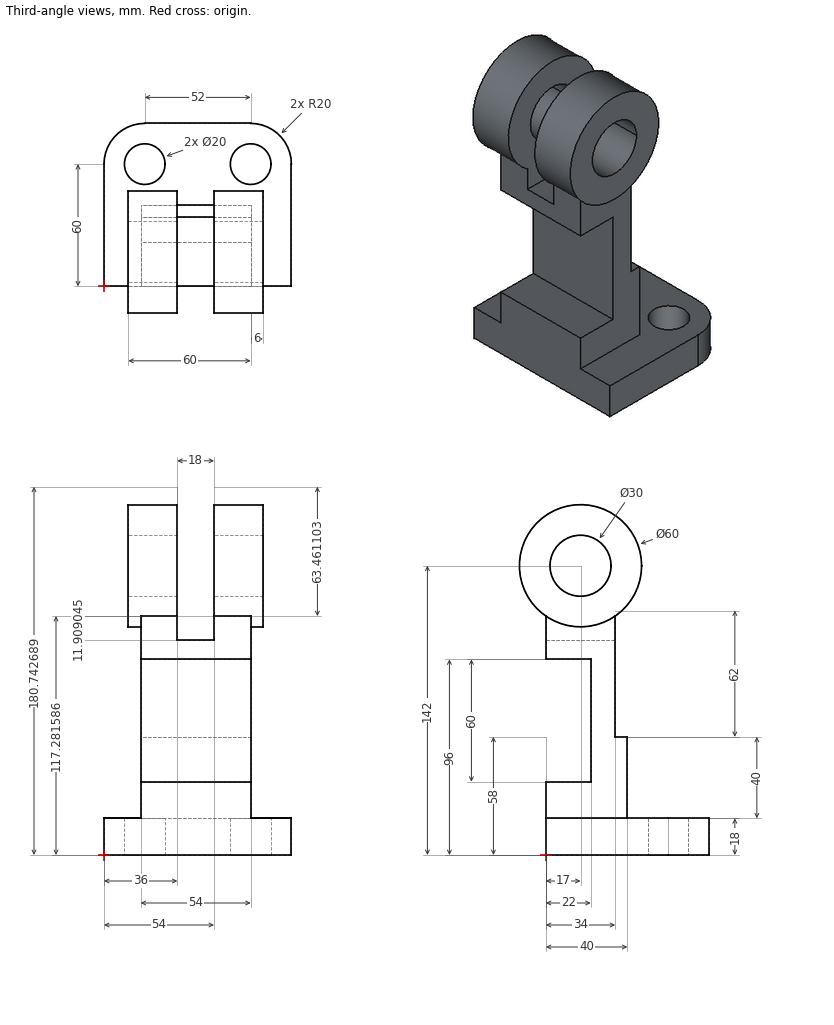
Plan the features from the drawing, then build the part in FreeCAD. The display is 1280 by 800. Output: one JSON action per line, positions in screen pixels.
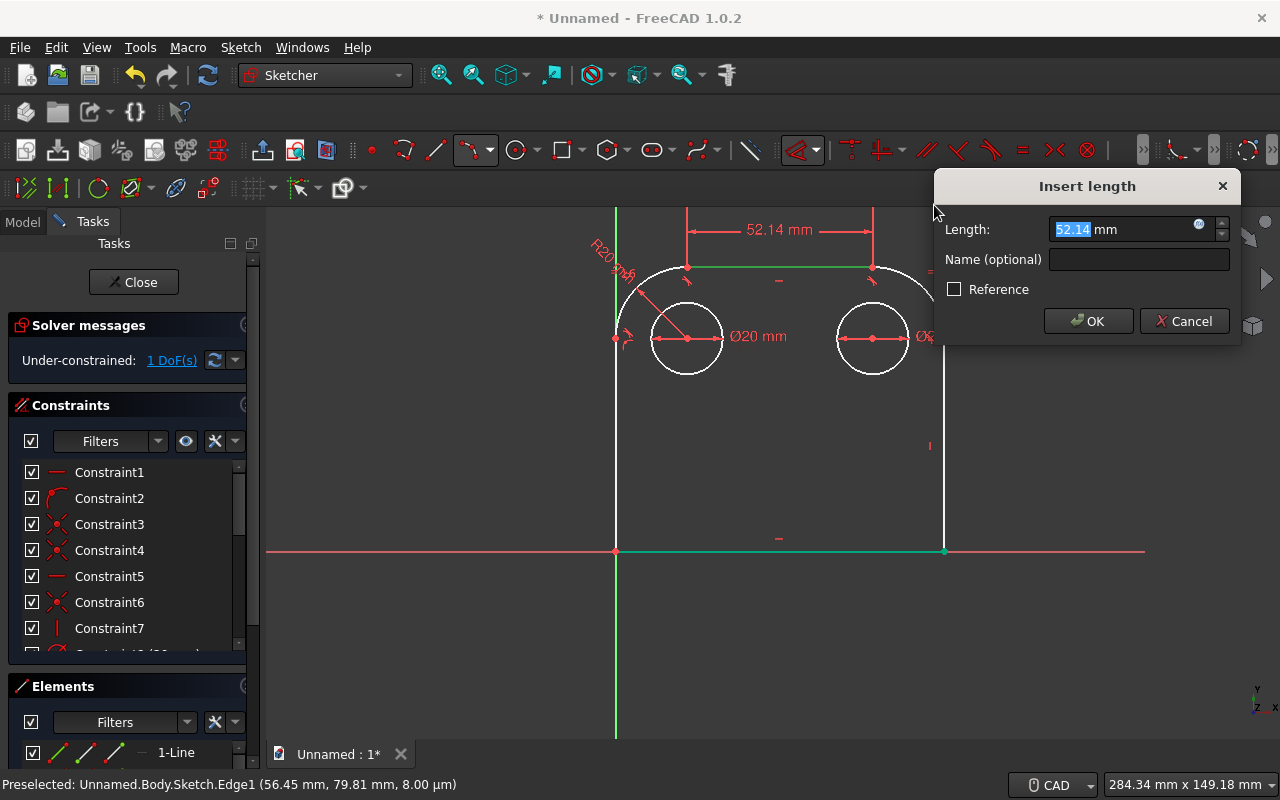
{"action": "type", "text": "52"}
{"action": "key", "text": "Return"}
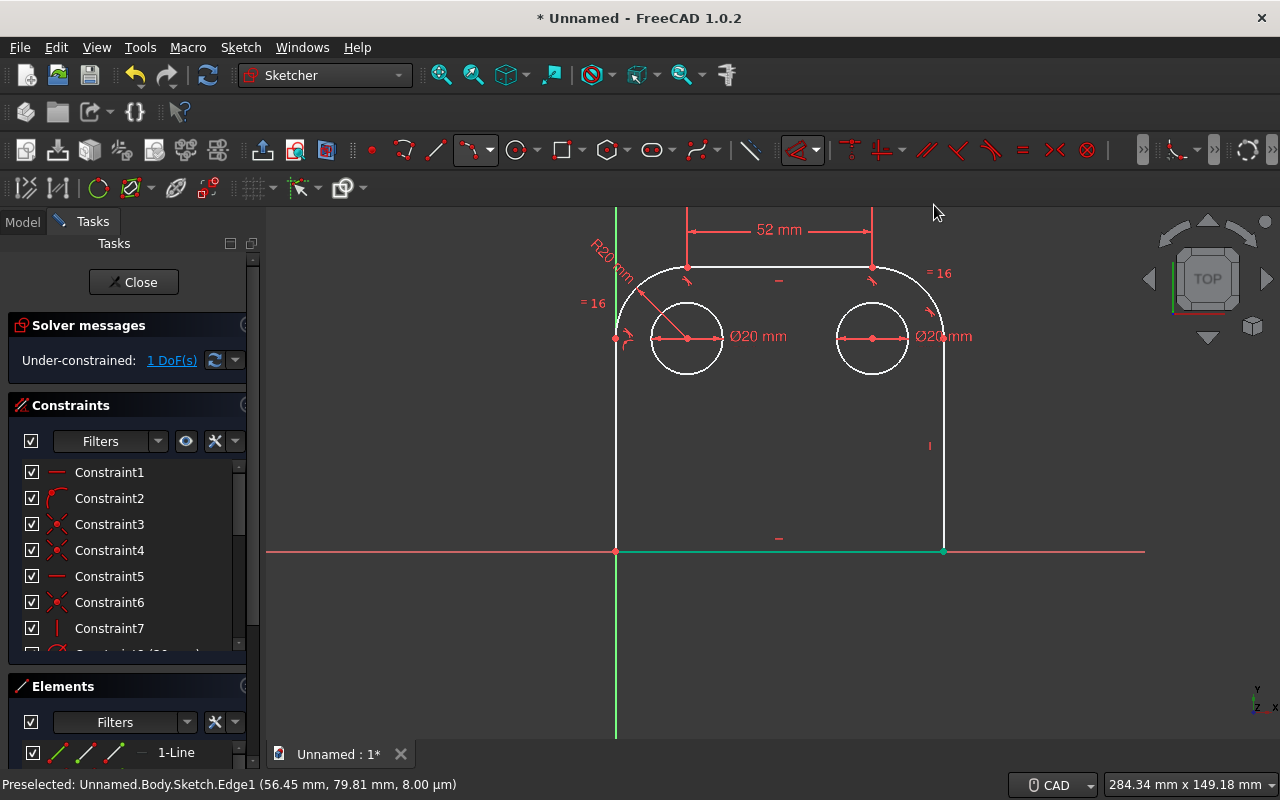
{"action": "left_click", "coordinate": [616, 402]}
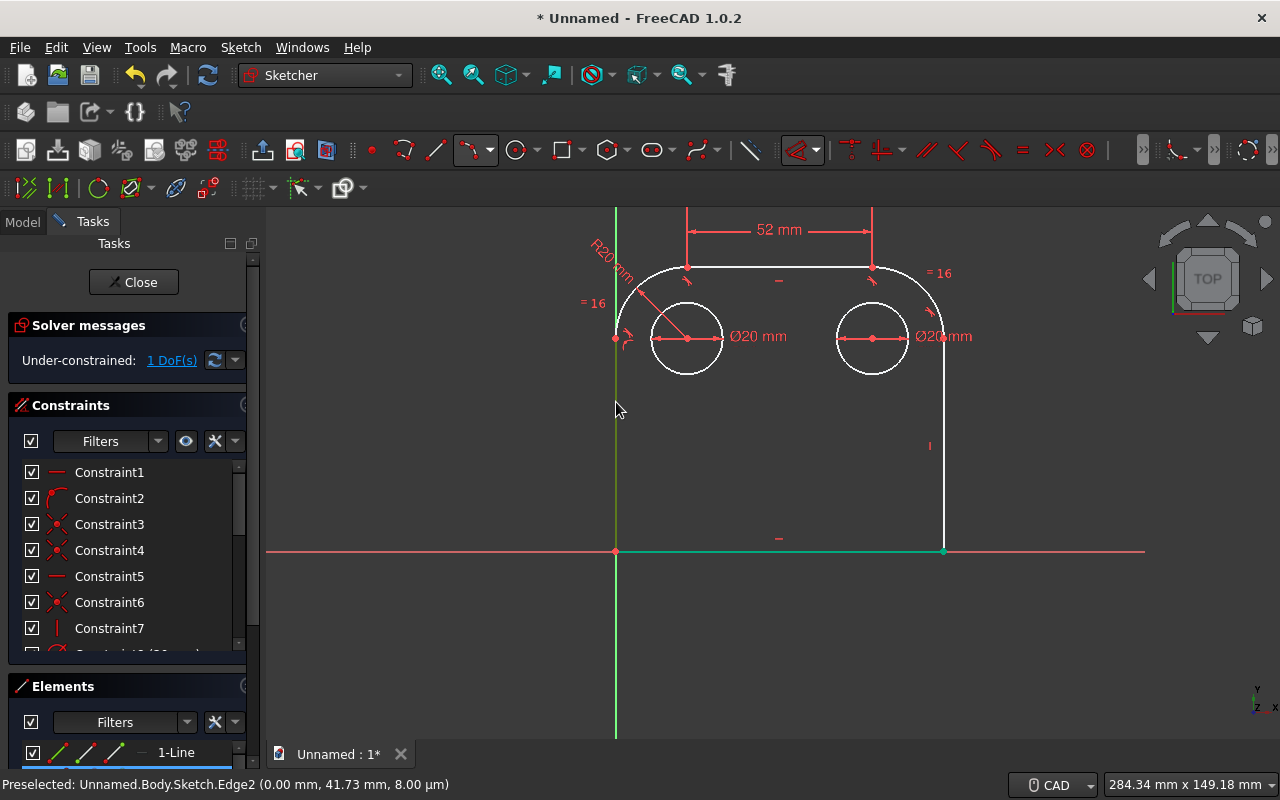
{"action": "key", "text": "i"}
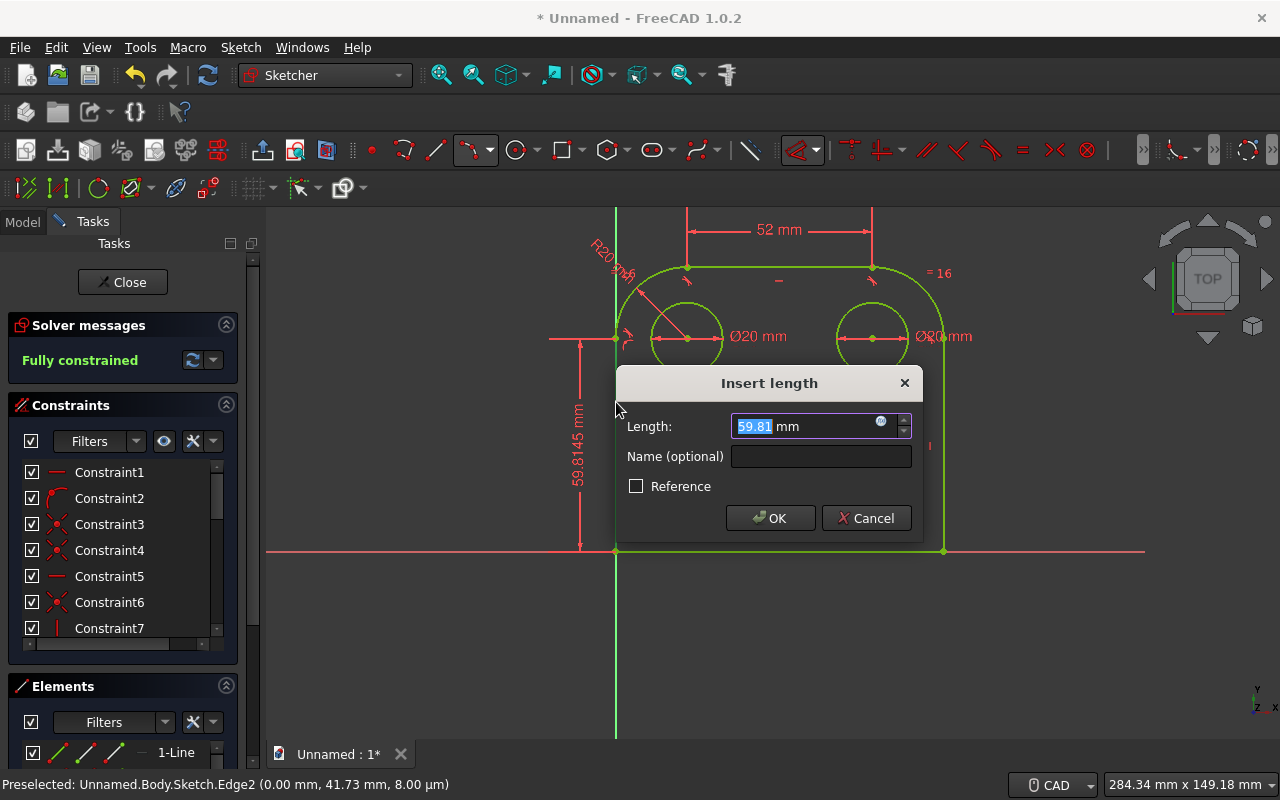
{"action": "type", "text": "60"}
{"action": "key", "text": "Return"}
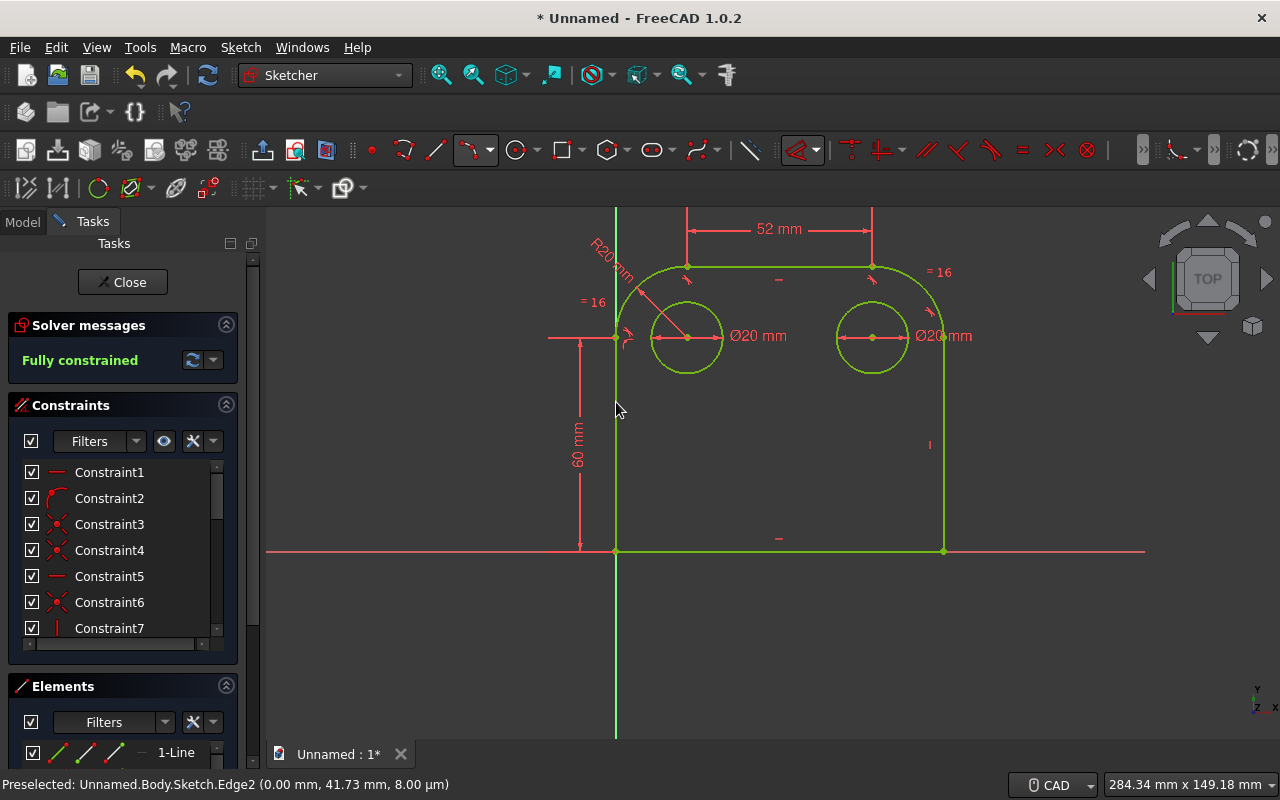
{"action": "left_click", "coordinate": [123, 282]}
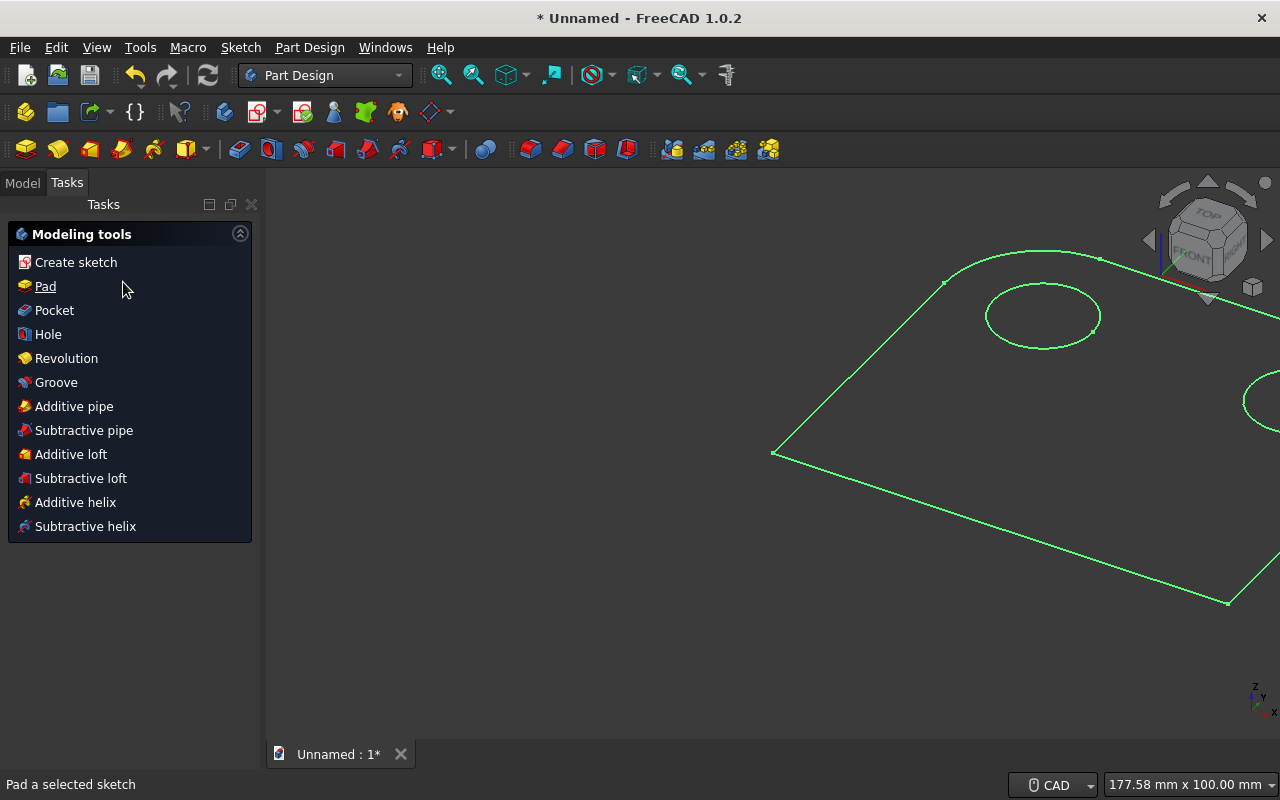
{"action": "left_click", "coordinate": [26, 150]}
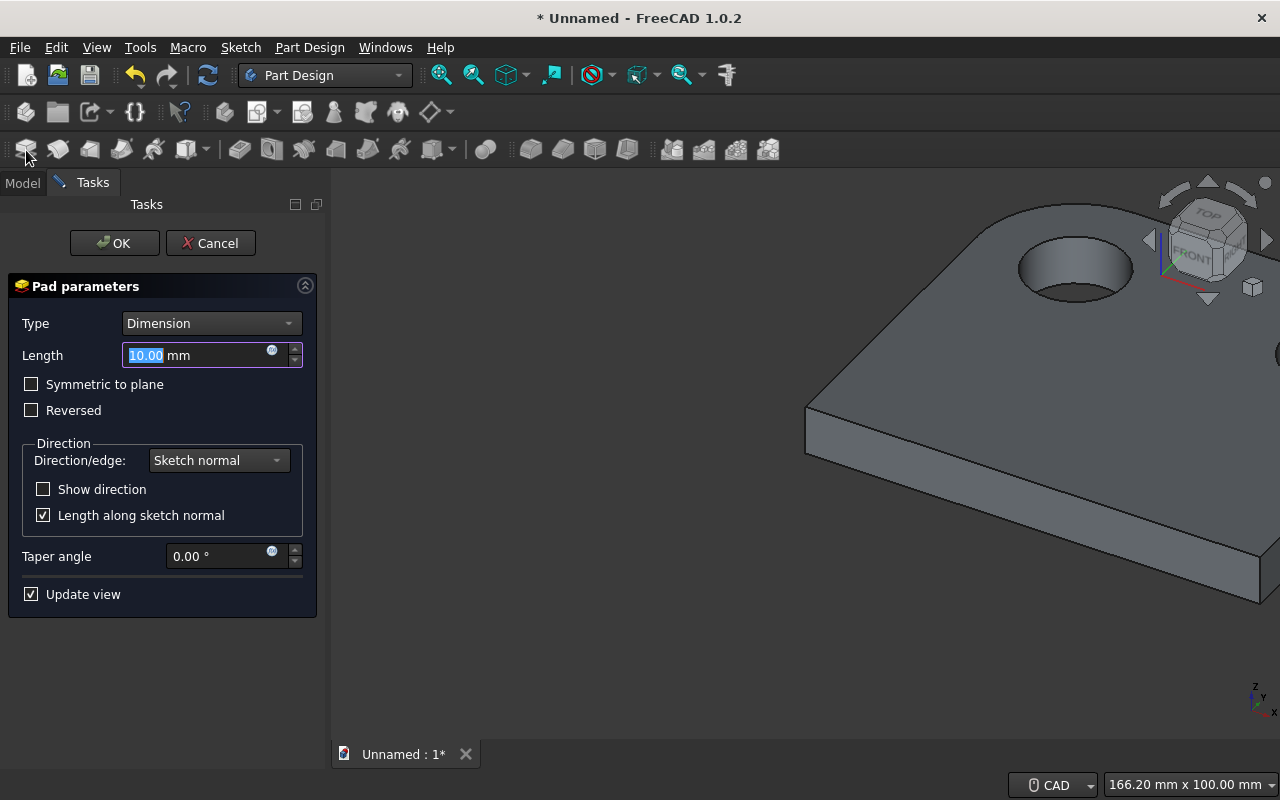
{"action": "type", "text": "18"}
{"action": "key", "text": "Tab"}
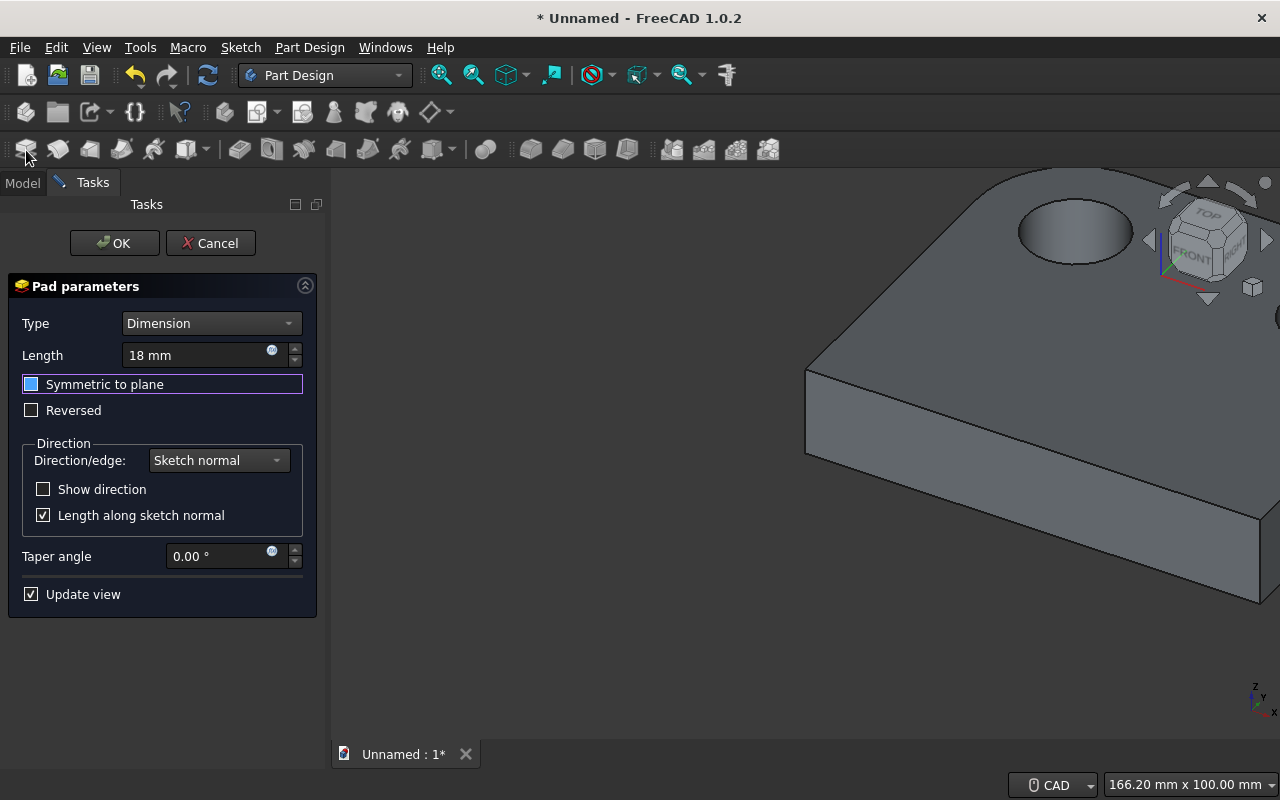
{"action": "left_click", "coordinate": [115, 243]}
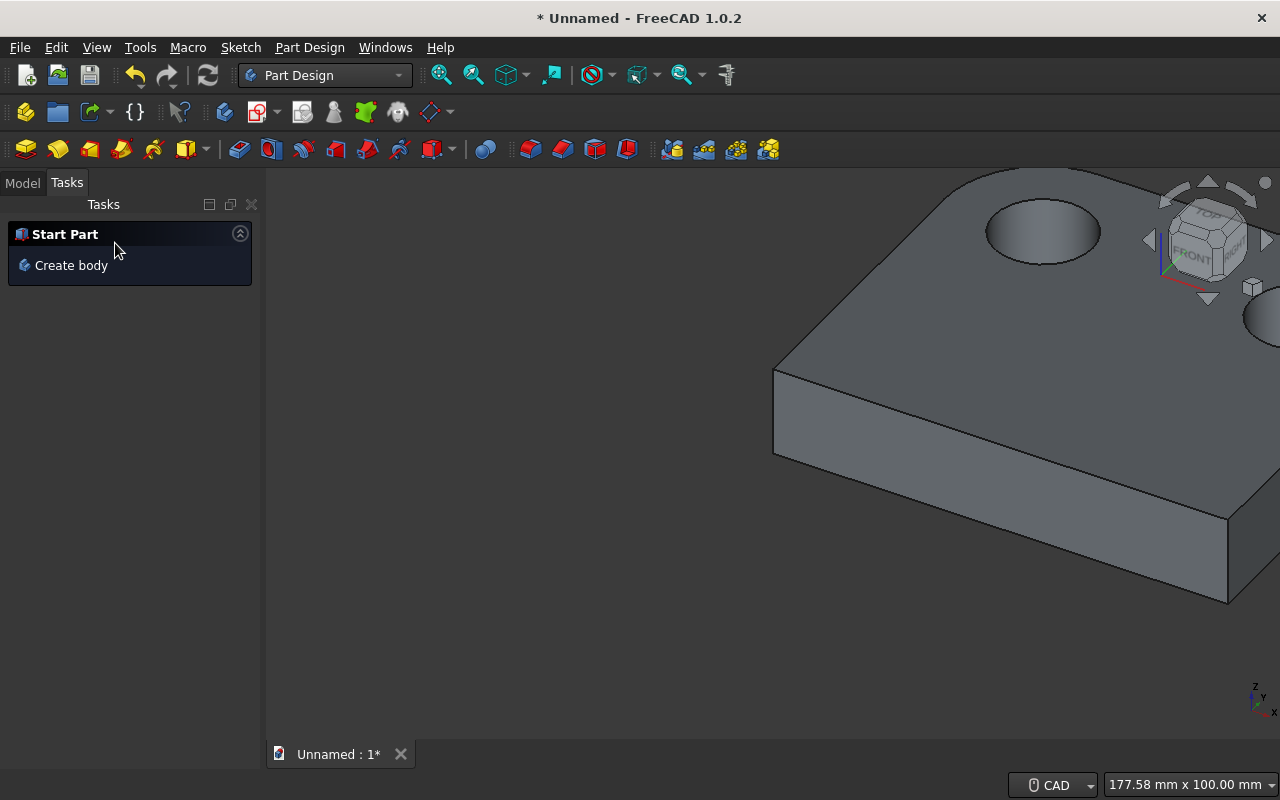
{"action": "left_click", "coordinate": [442, 76]}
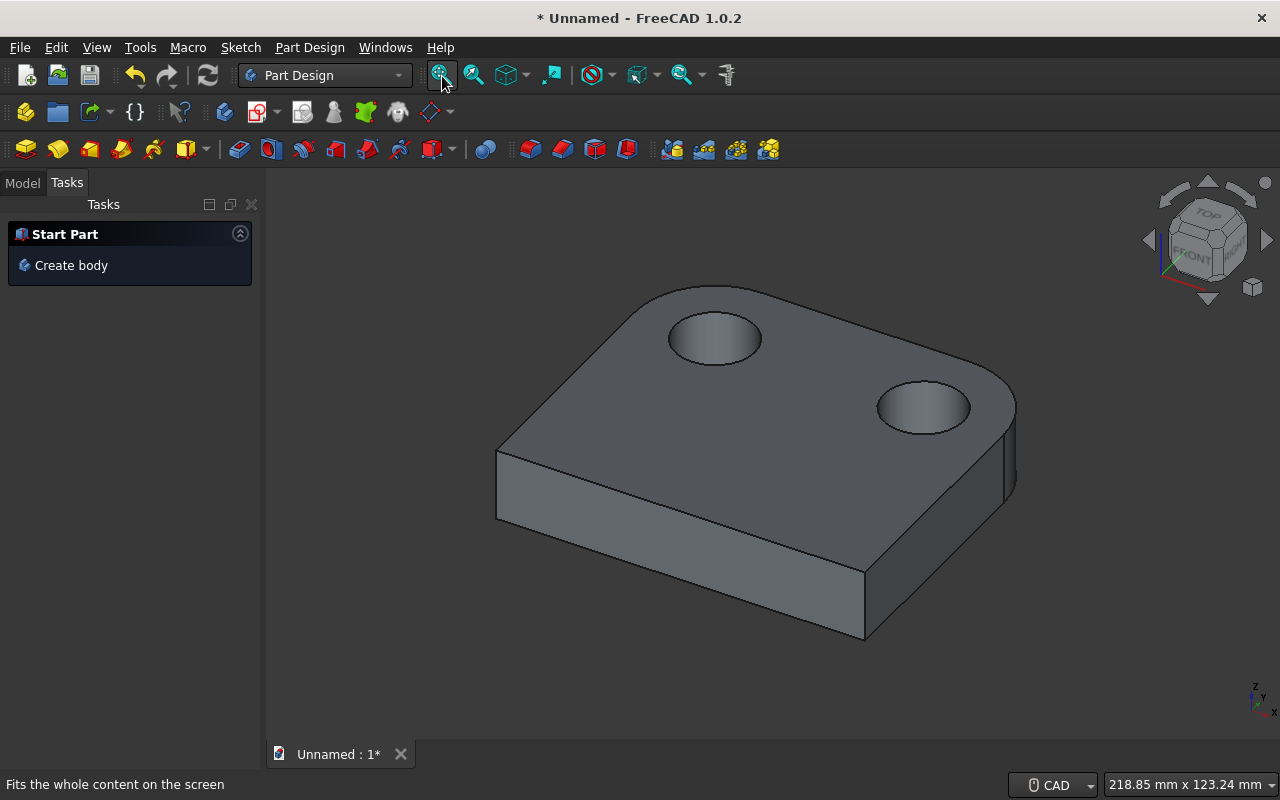
{"action": "left_click", "coordinate": [23, 182]}